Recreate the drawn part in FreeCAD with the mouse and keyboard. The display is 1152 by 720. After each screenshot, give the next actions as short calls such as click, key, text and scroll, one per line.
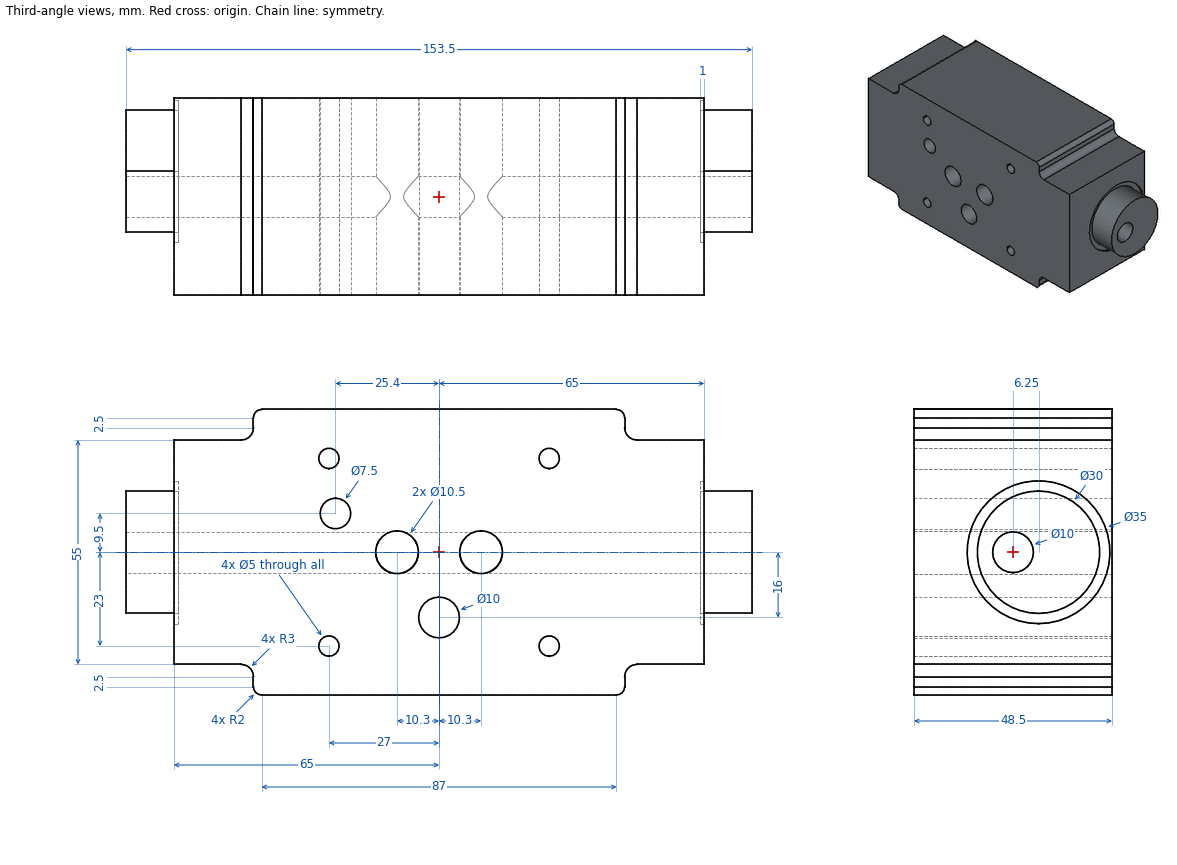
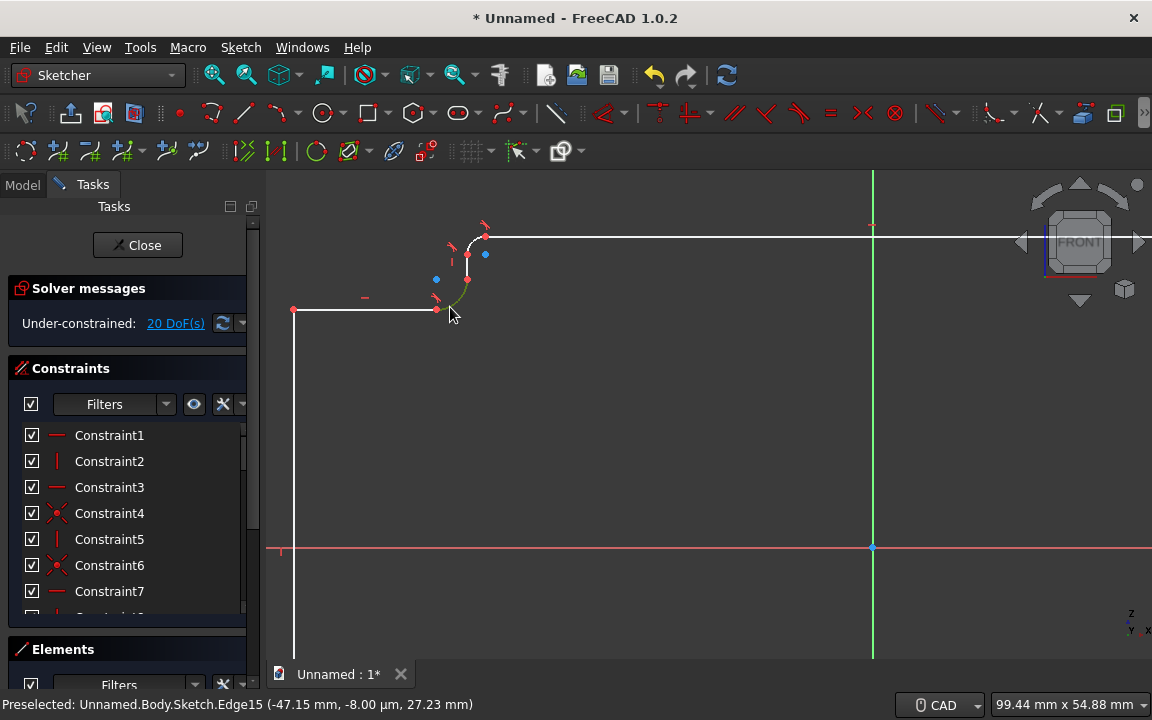
scroll(451, 306, down, 4)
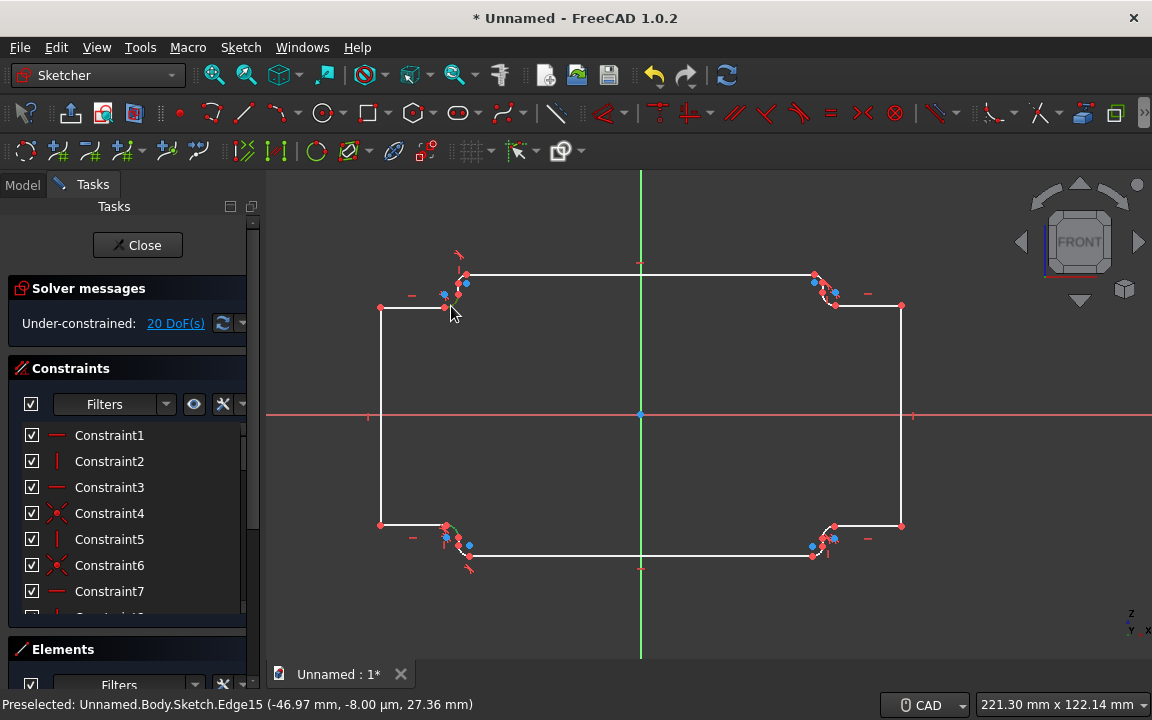
scroll(824, 299, up, 5)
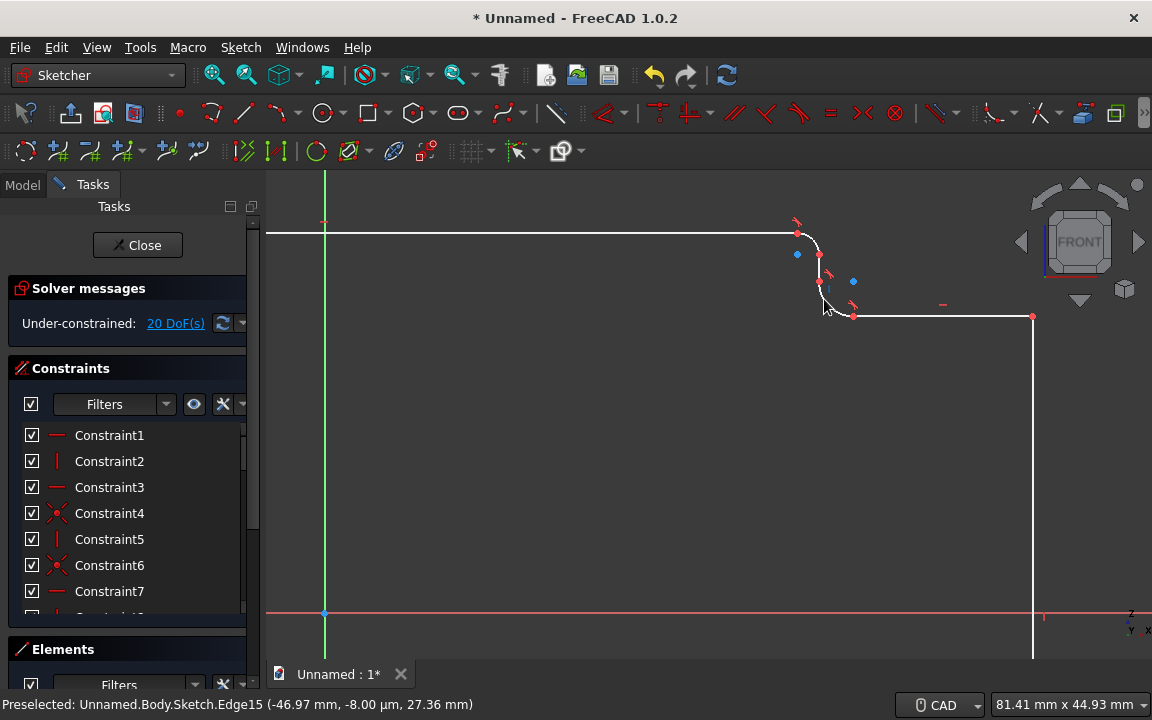
click(823, 298)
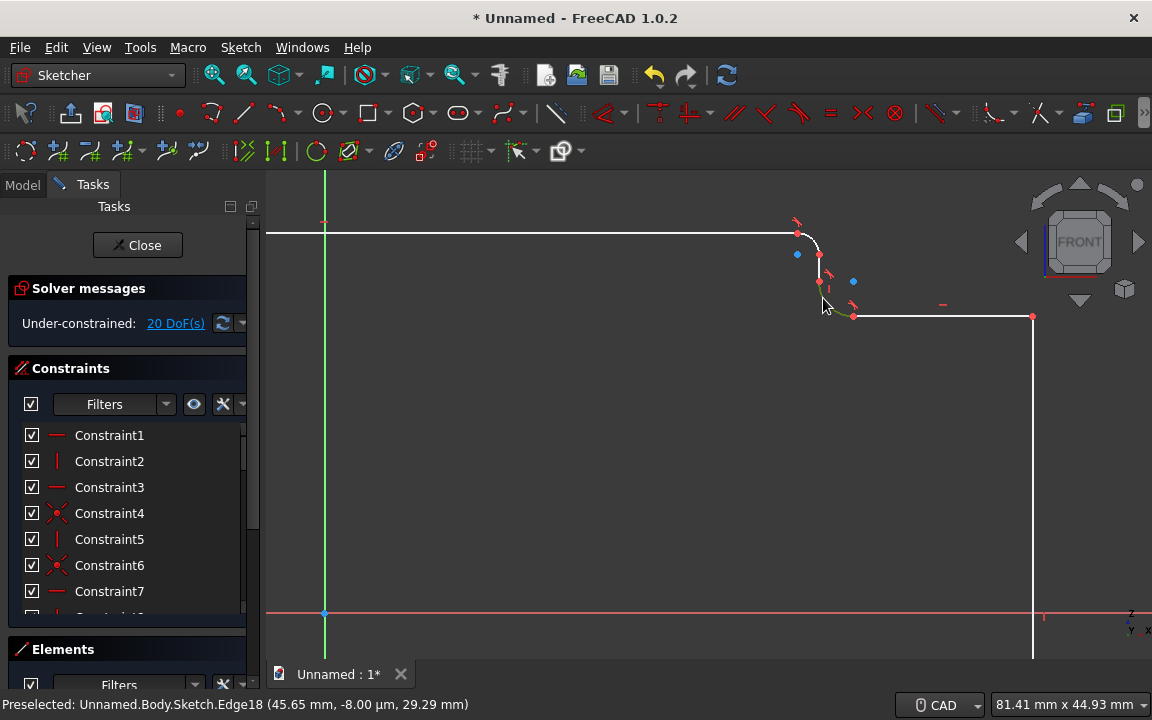
scroll(824, 299, down, 5)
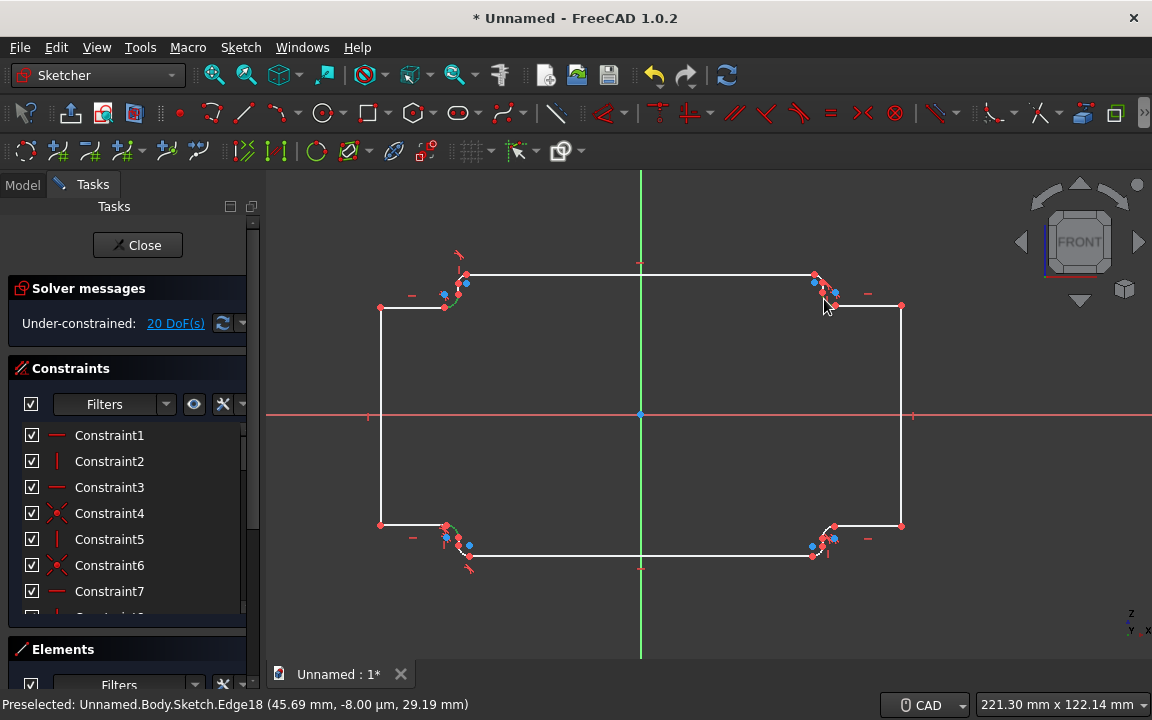
scroll(829, 527, up, 5)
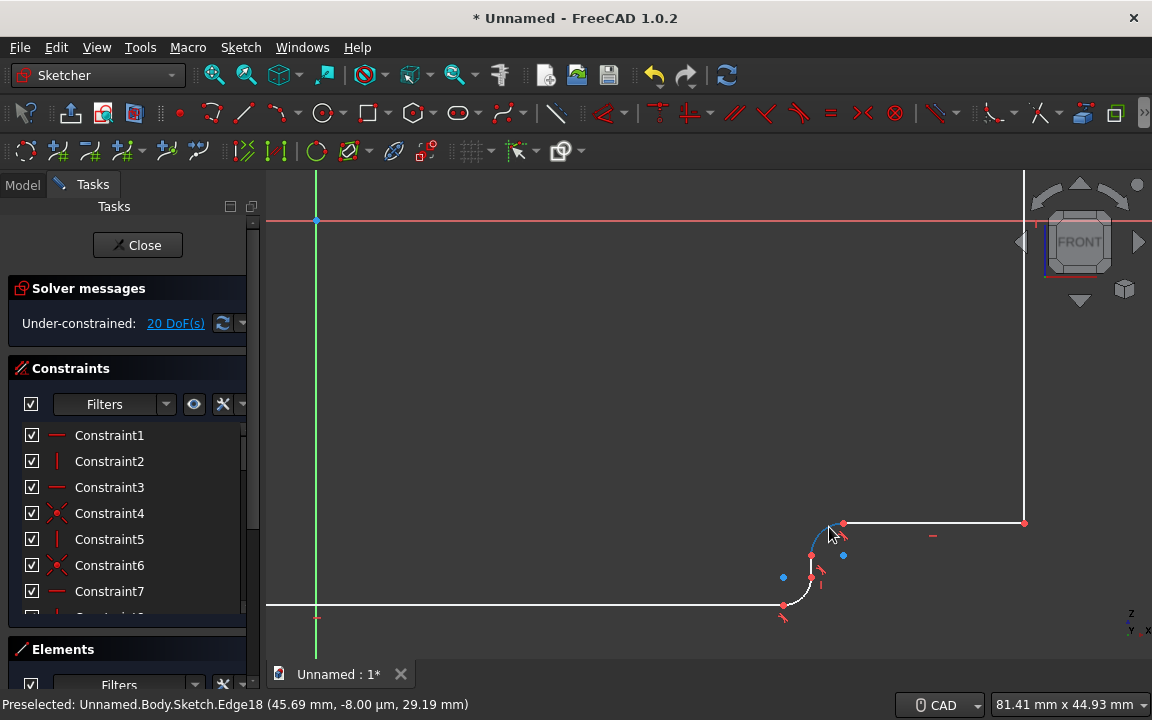
click(829, 527)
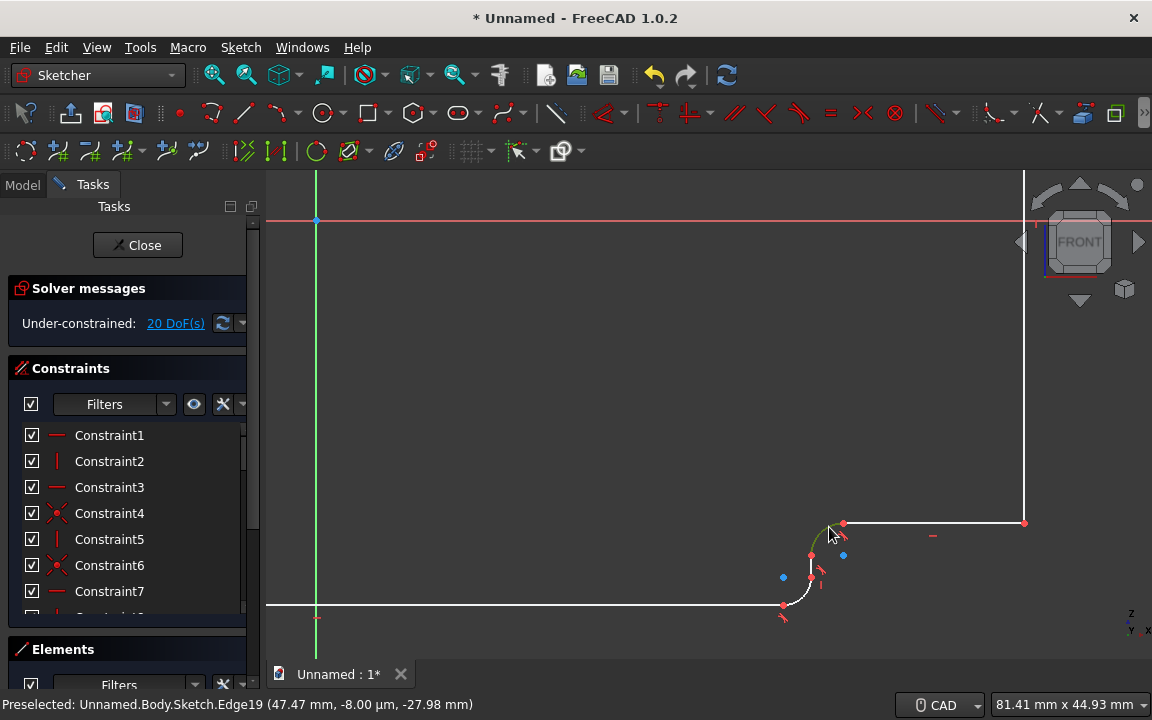
click(832, 114)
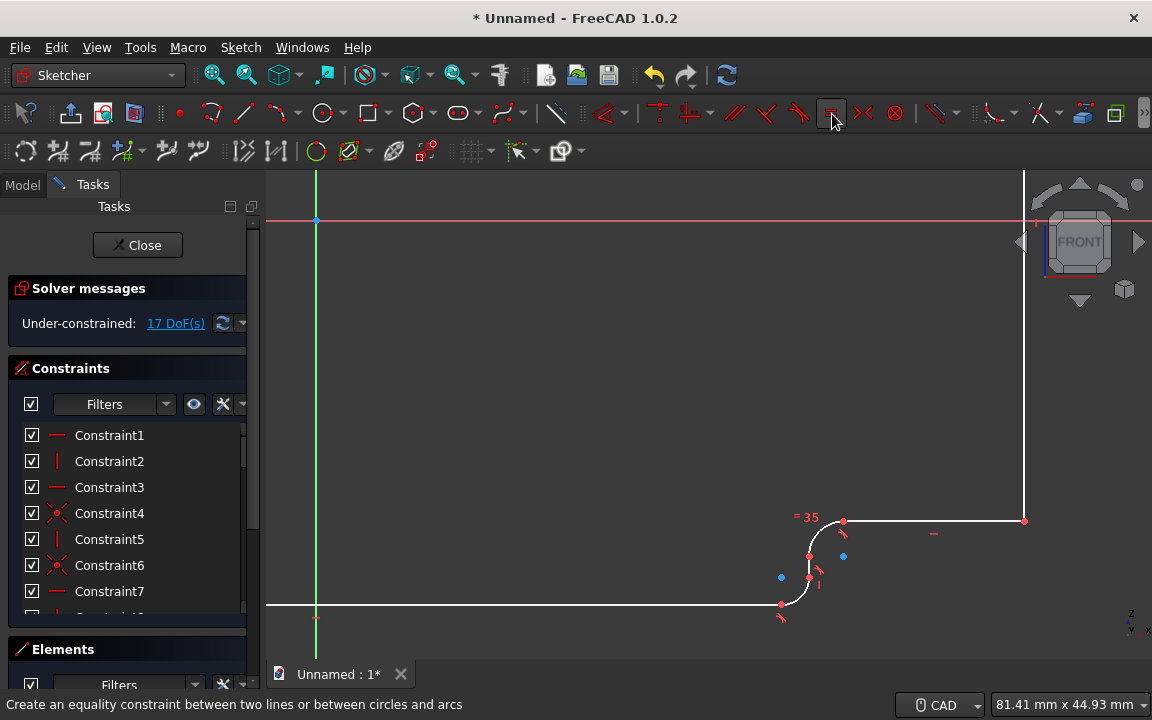
scroll(829, 527, down, 5)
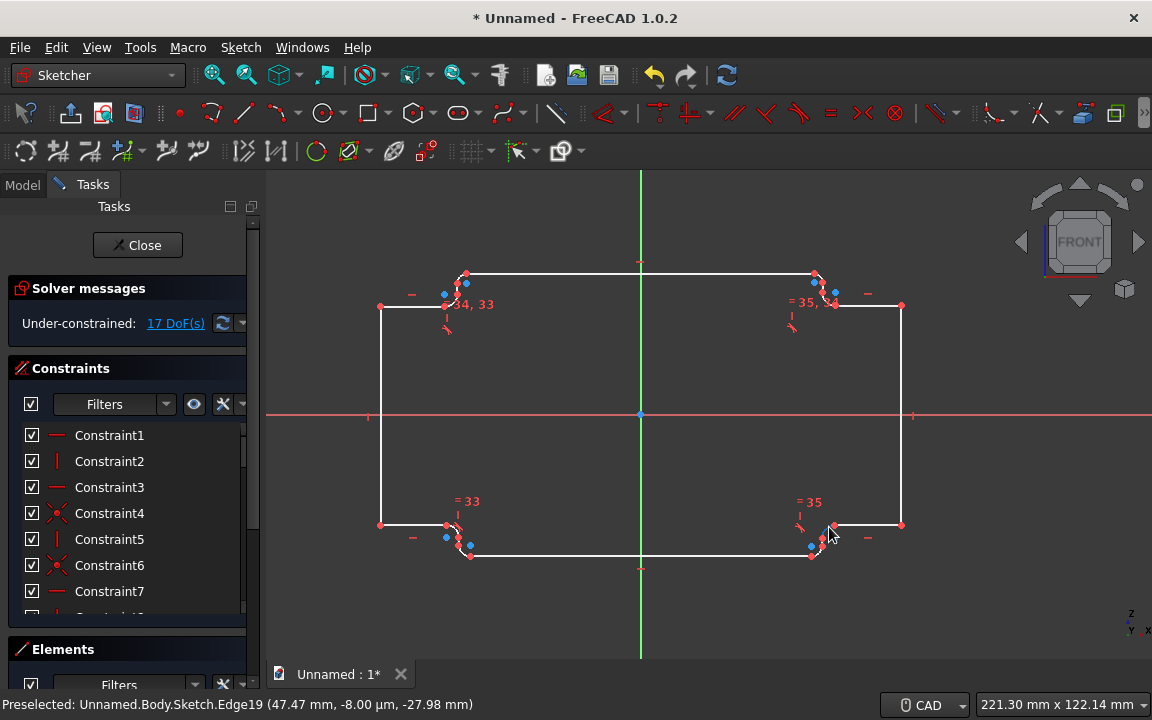
scroll(460, 550, up, 5)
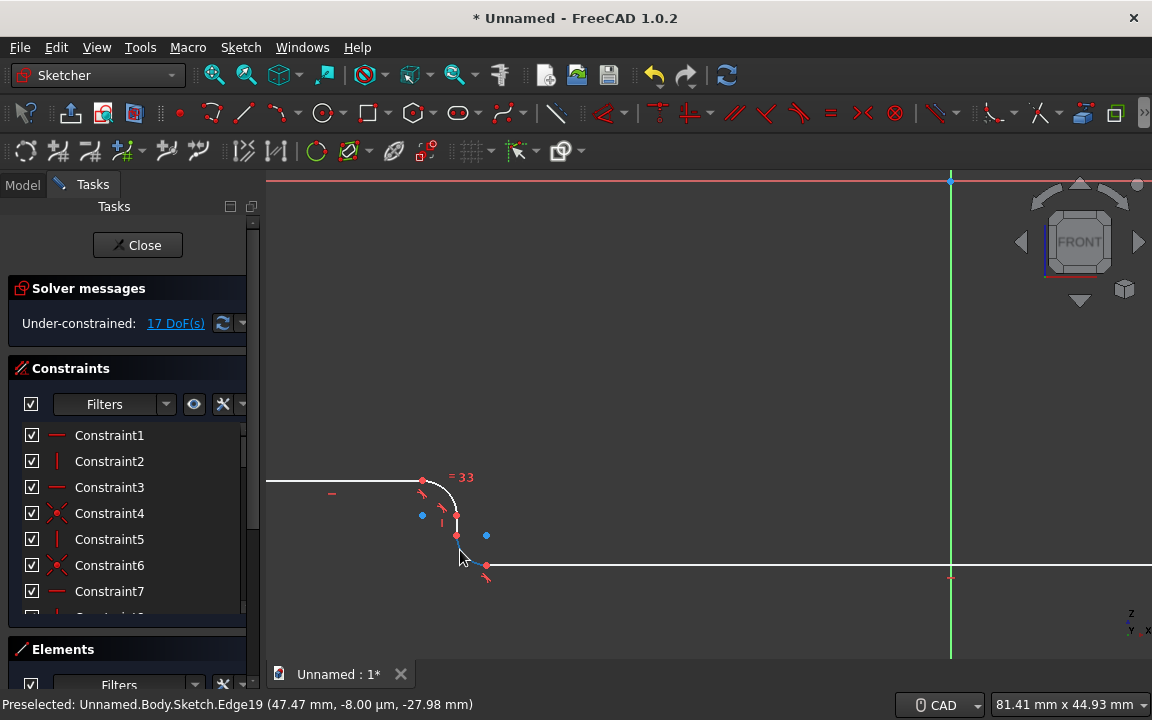
click(460, 549)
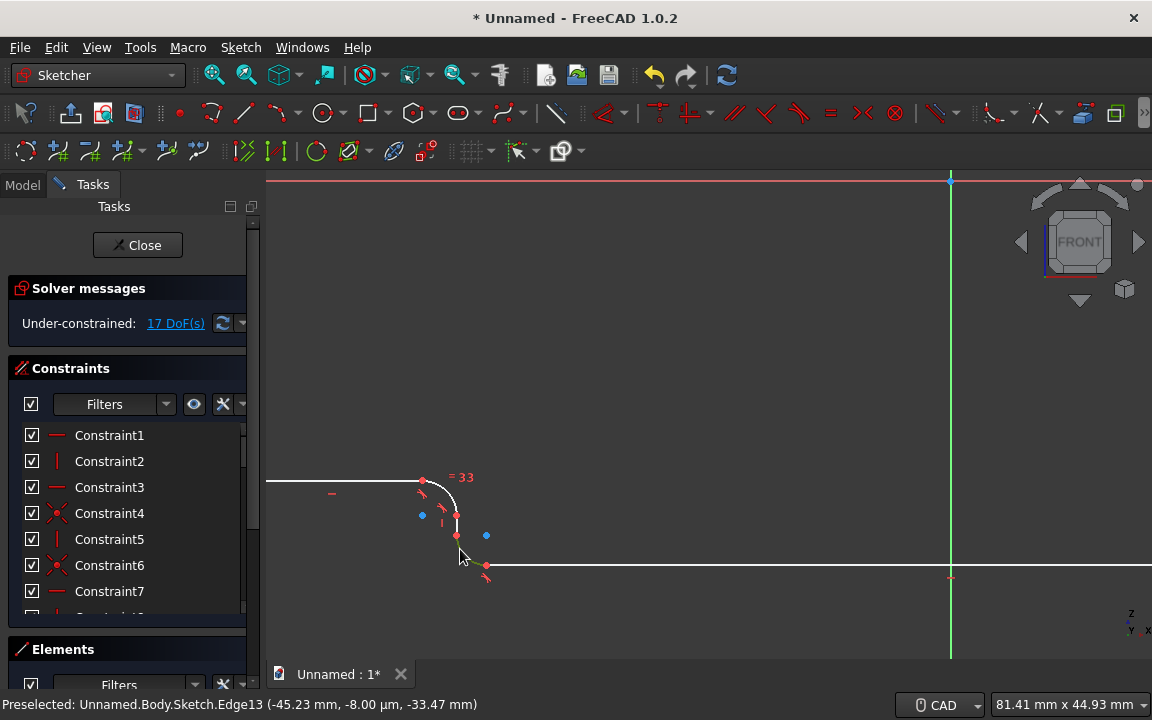
scroll(460, 550, down, 5)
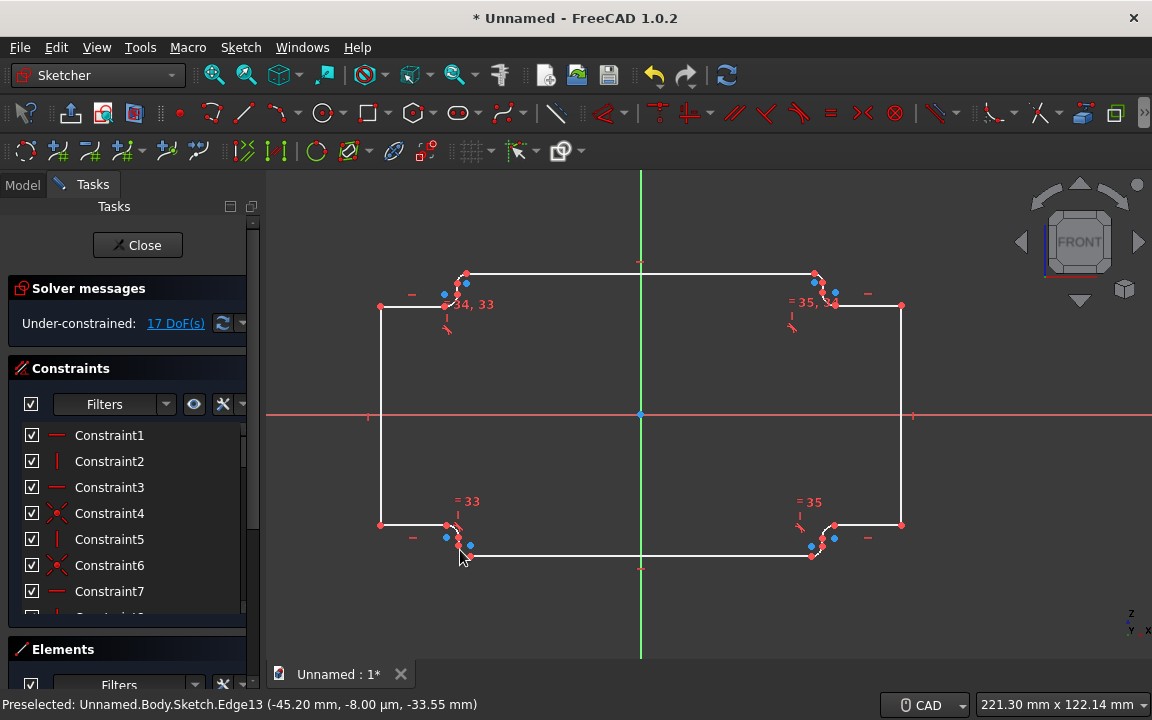
scroll(462, 275, up, 6)